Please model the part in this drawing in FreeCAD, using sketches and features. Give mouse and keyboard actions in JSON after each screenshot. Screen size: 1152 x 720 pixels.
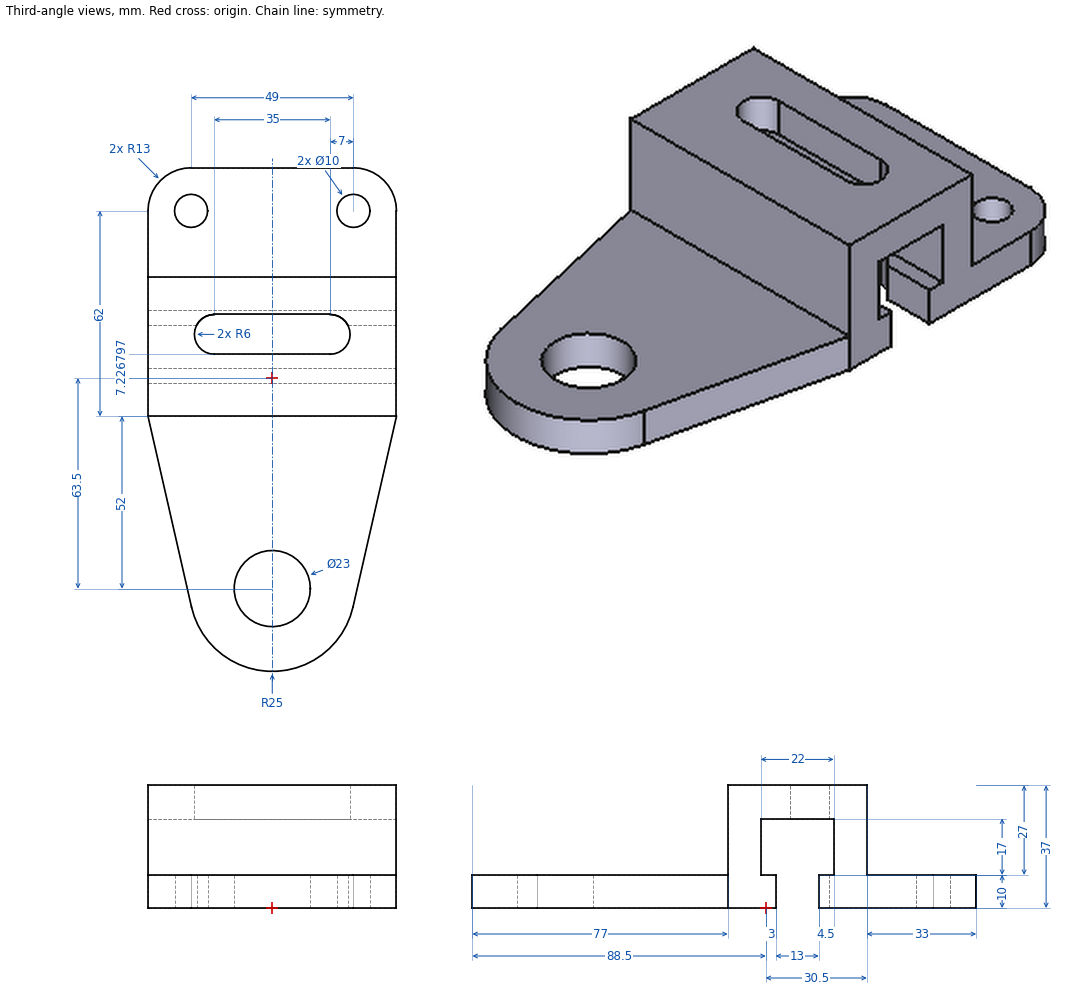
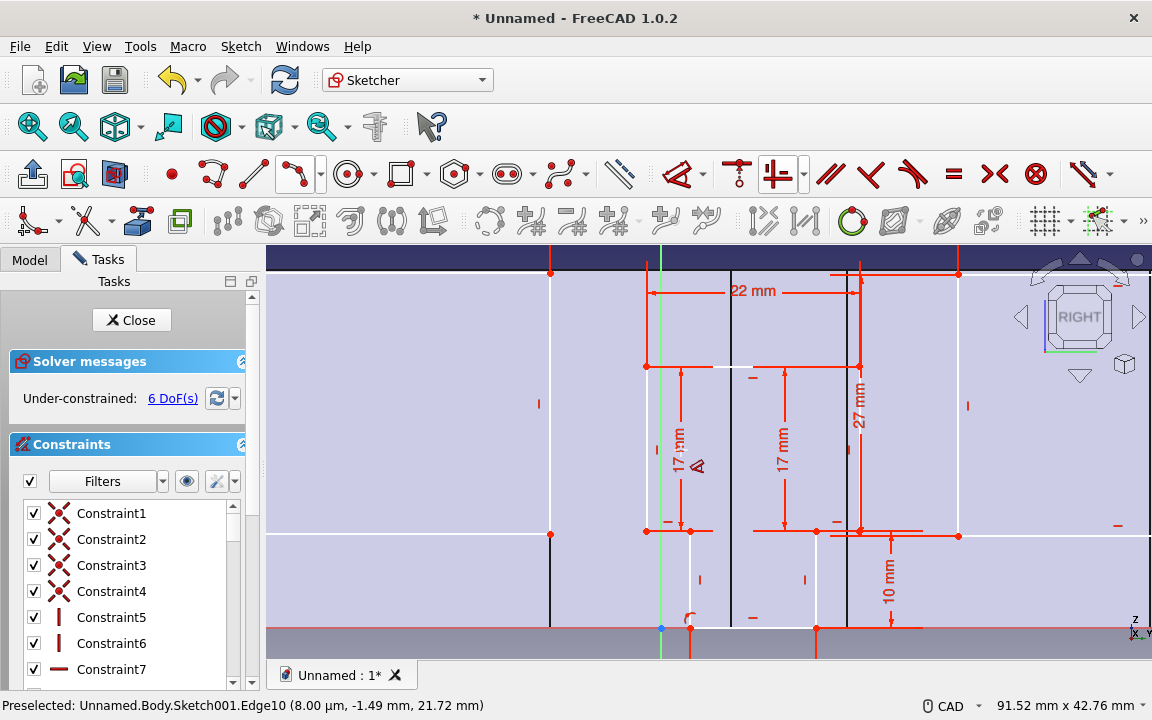
{"action": "scroll", "coordinate": [690, 628], "scroll_direction": "up", "scroll_amount": 2}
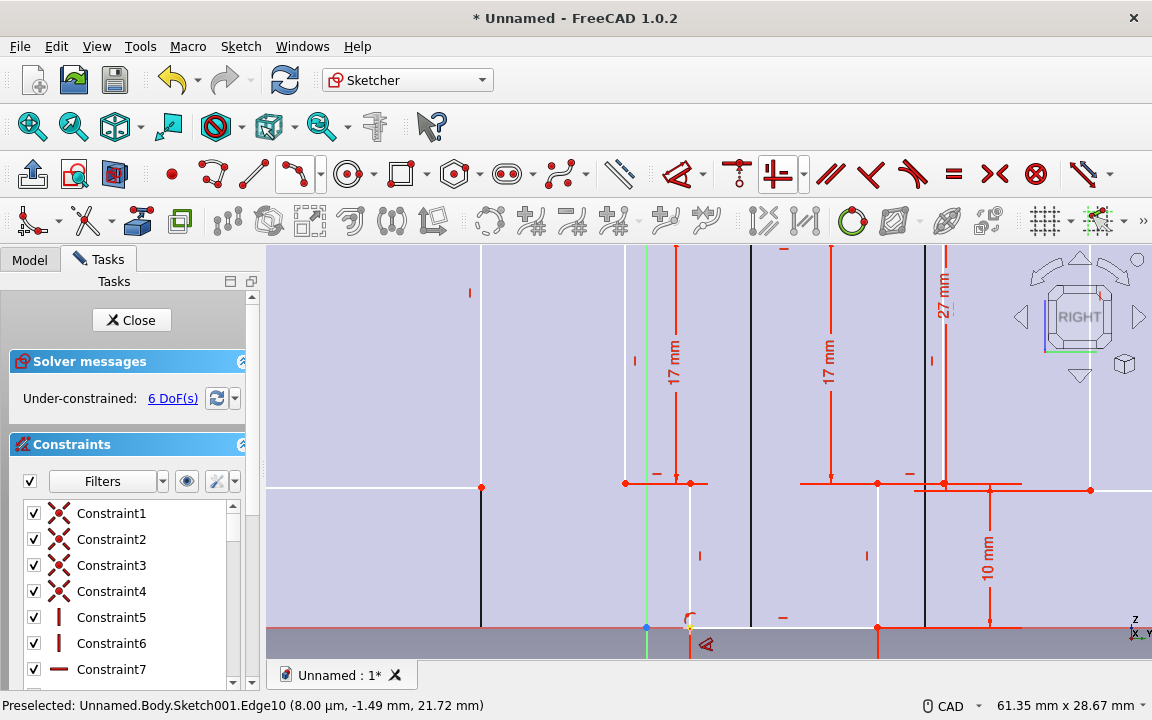
{"action": "left_click", "coordinate": [690, 628]}
{"action": "left_click", "coordinate": [668, 594]}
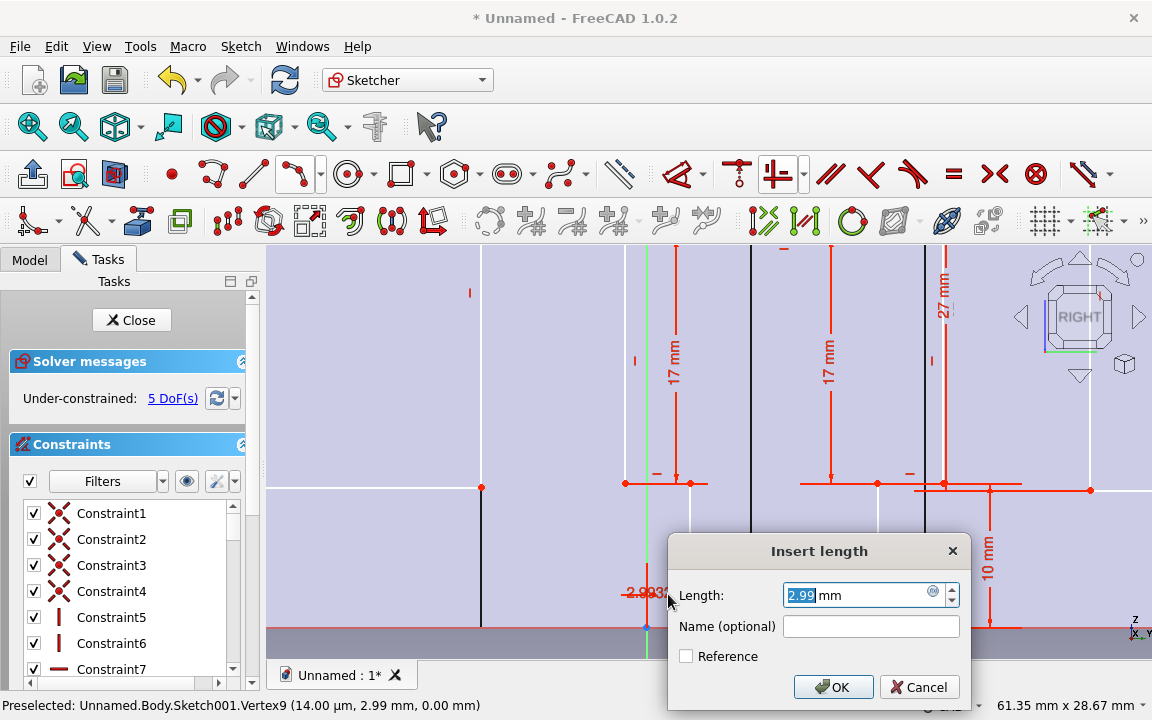
{"action": "type", "text": "3"}
{"action": "key", "text": "Return"}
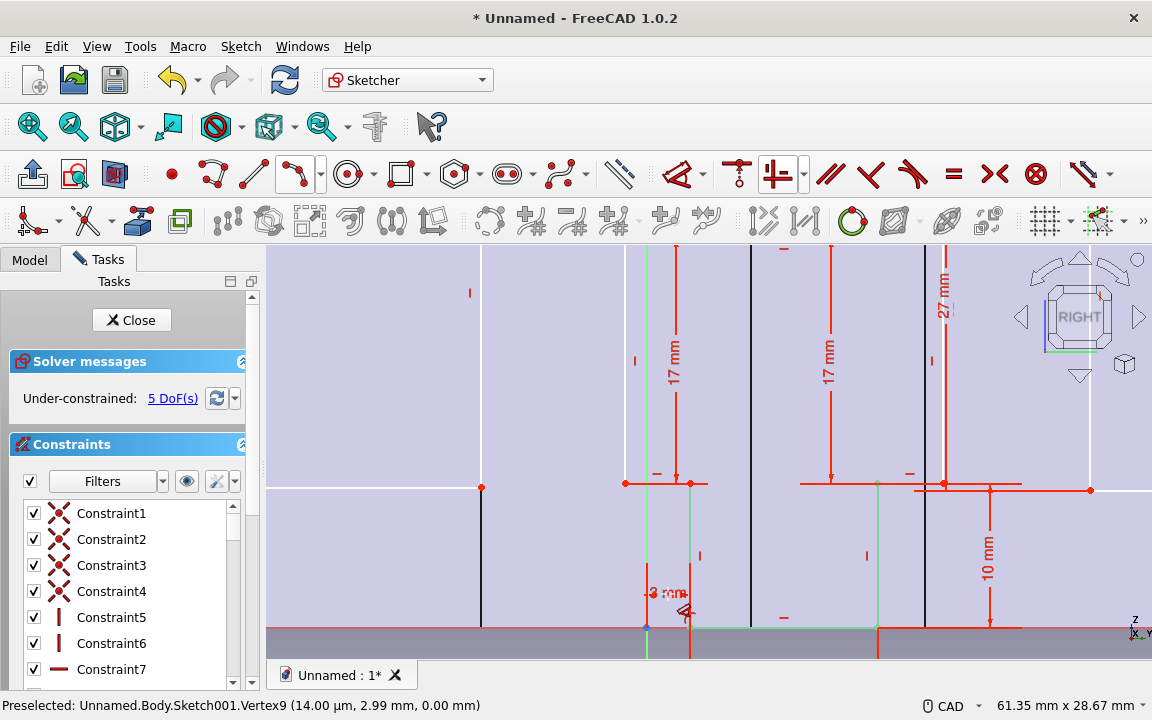
{"action": "left_click", "coordinate": [897, 484]}
{"action": "left_click", "coordinate": [911, 518]}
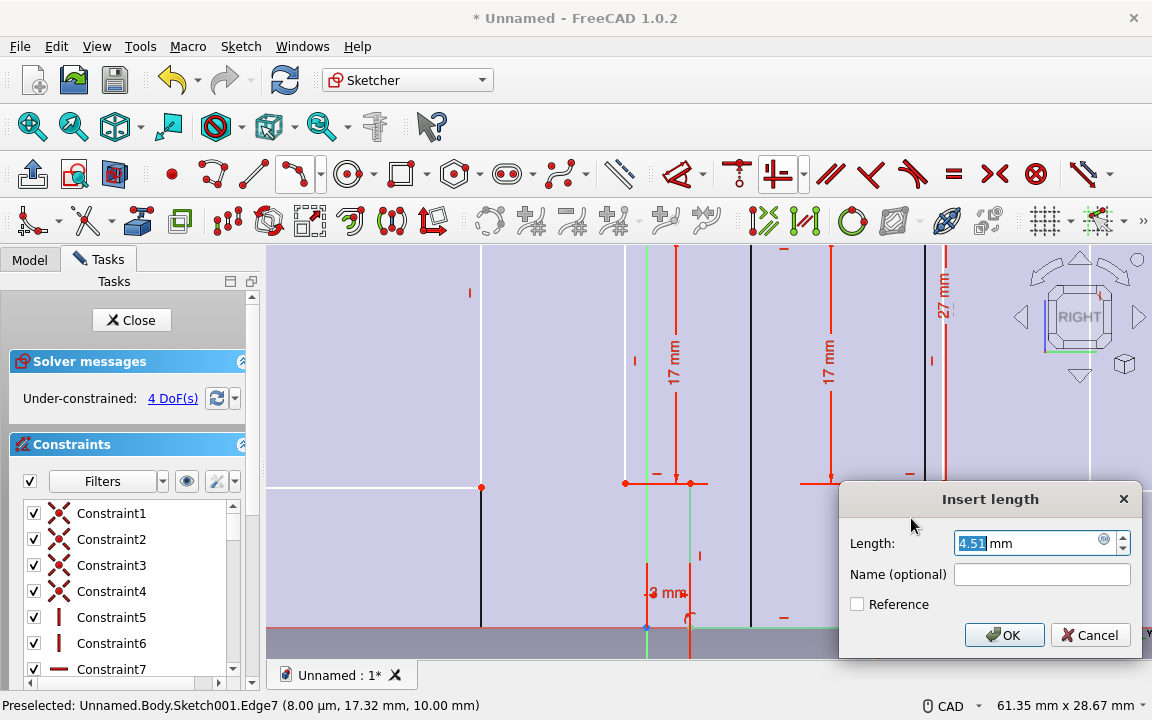
{"action": "type", "text": "4.5"}
{"action": "key", "text": "Return"}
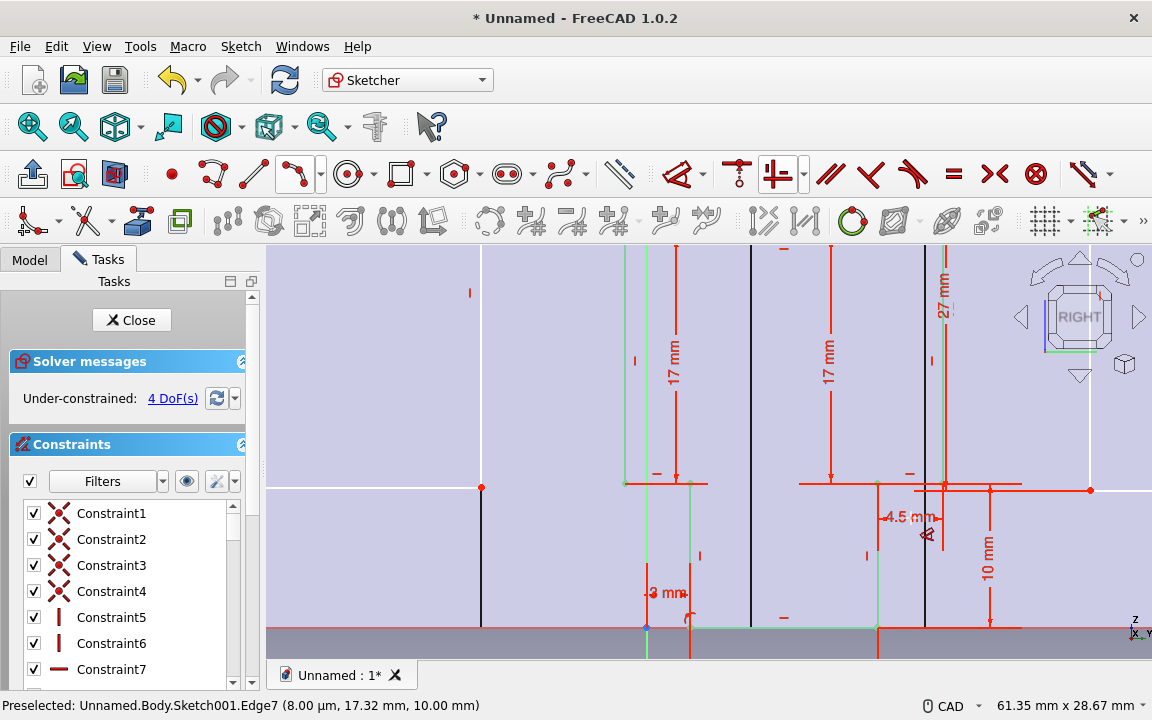
{"action": "scroll", "coordinate": [685, 475], "scroll_direction": "down", "scroll_amount": 8}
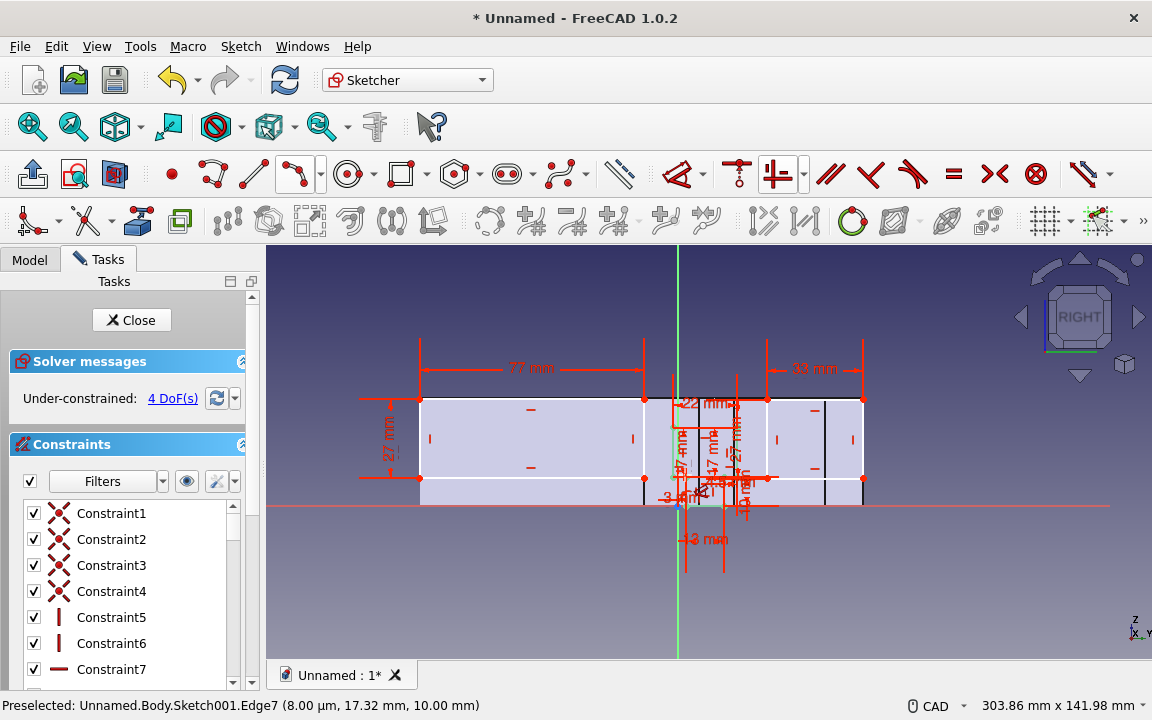
{"action": "left_click", "coordinate": [767, 400]}
{"action": "left_click", "coordinate": [801, 453]}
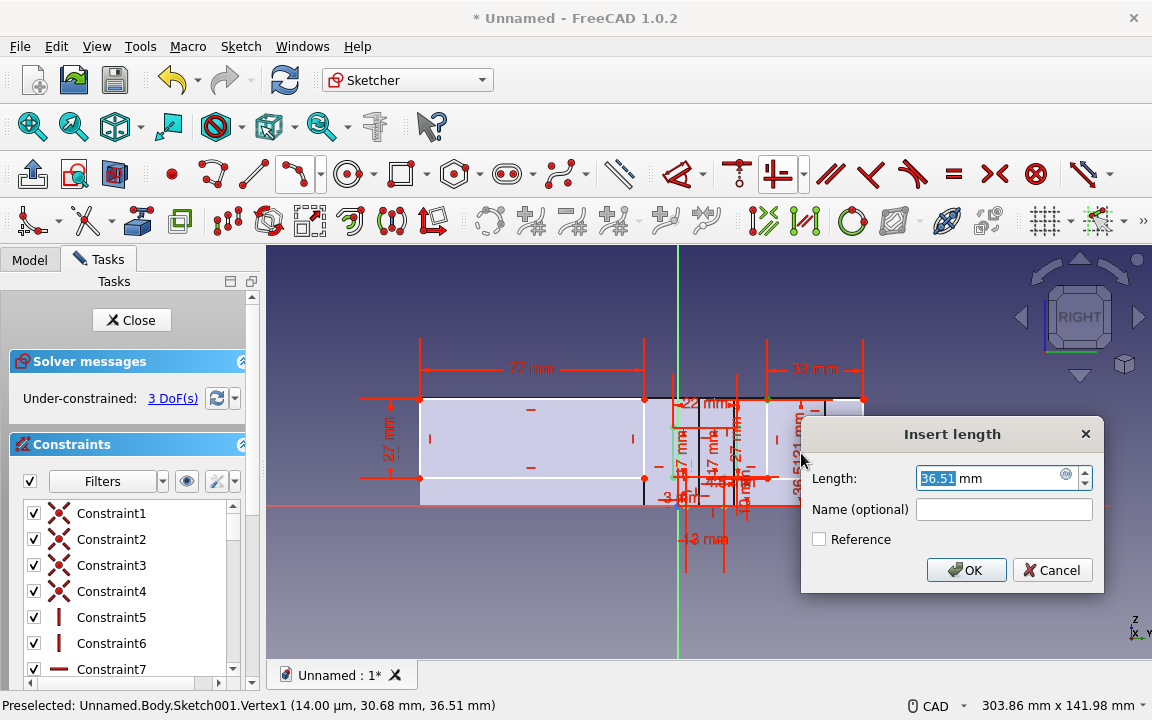
{"action": "type", "text": "37"}
{"action": "key", "text": "Return"}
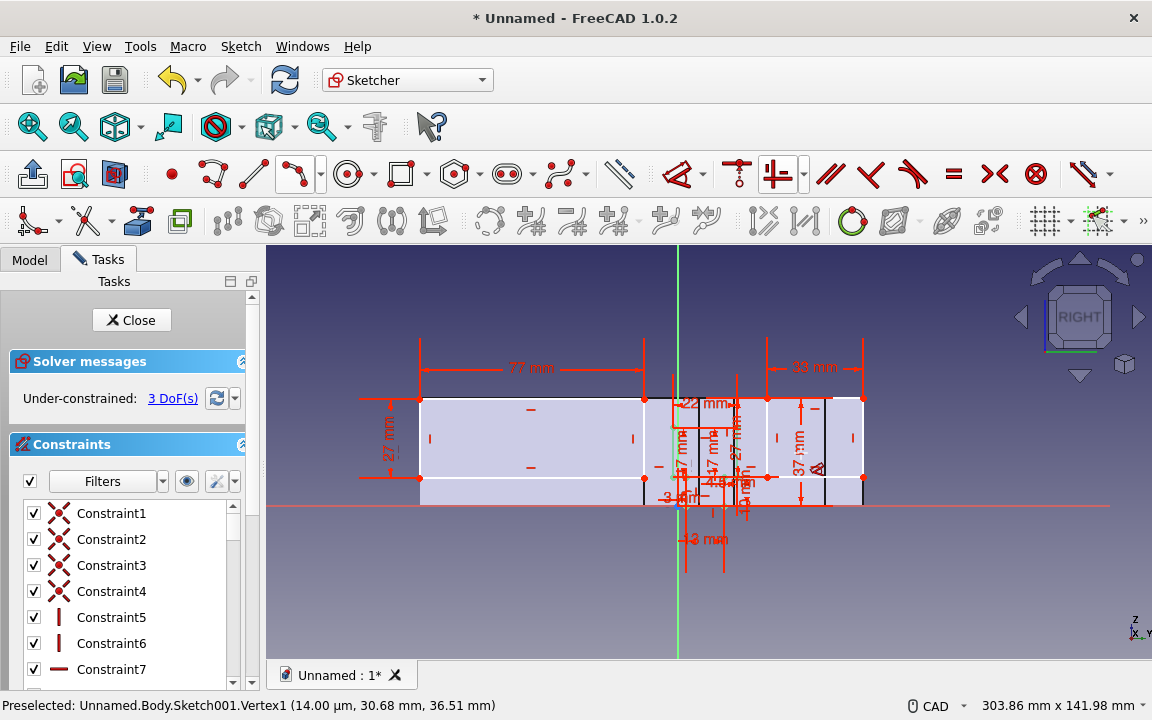
{"action": "left_click", "coordinate": [420, 399]}
{"action": "left_click", "coordinate": [386, 453]}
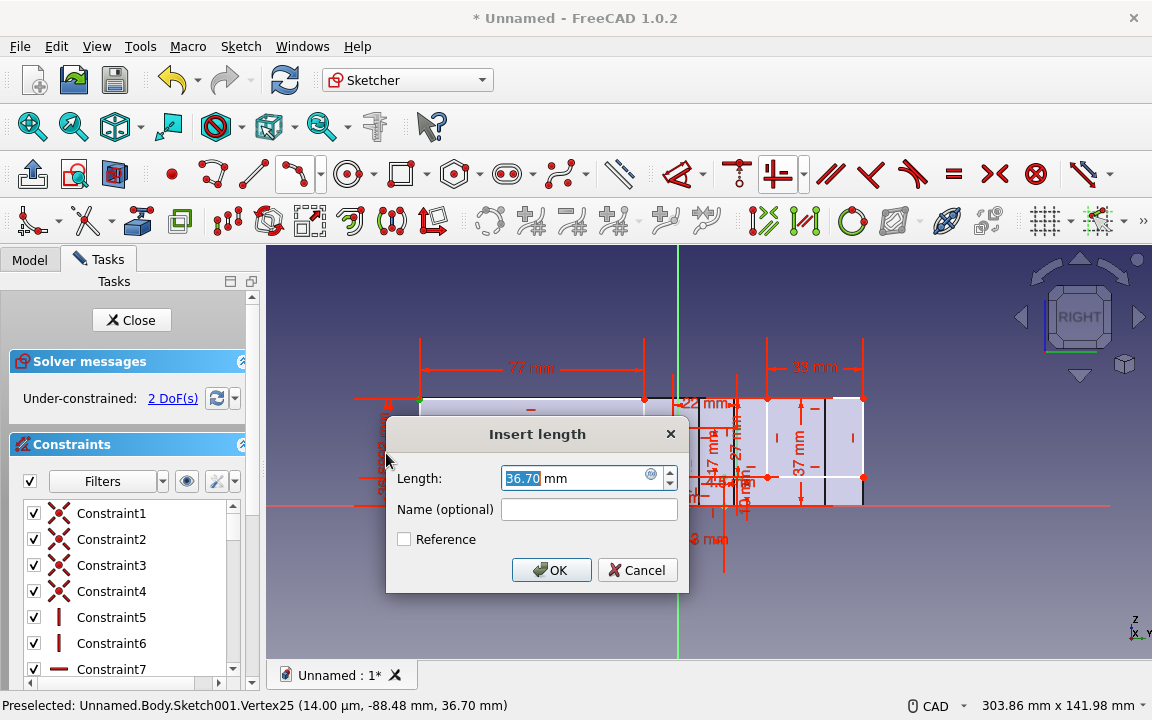
{"action": "type", "text": "37"}
{"action": "key", "text": "Return"}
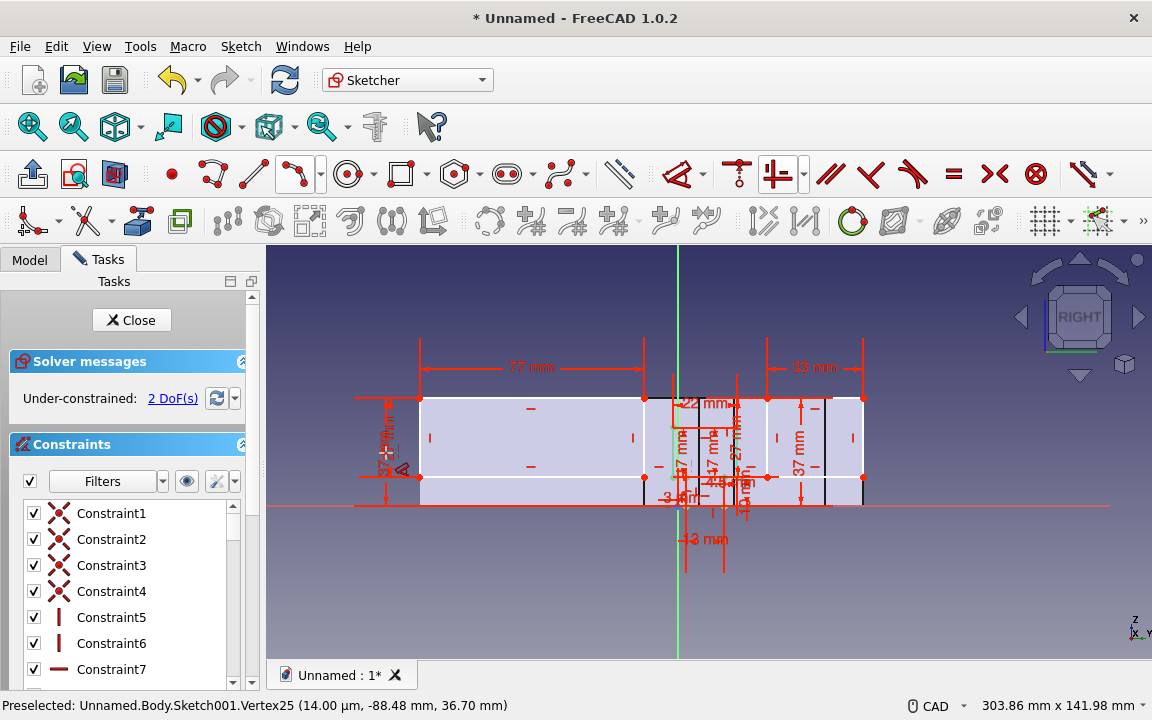
{"action": "left_click", "coordinate": [767, 398]}
{"action": "left_click", "coordinate": [722, 364]}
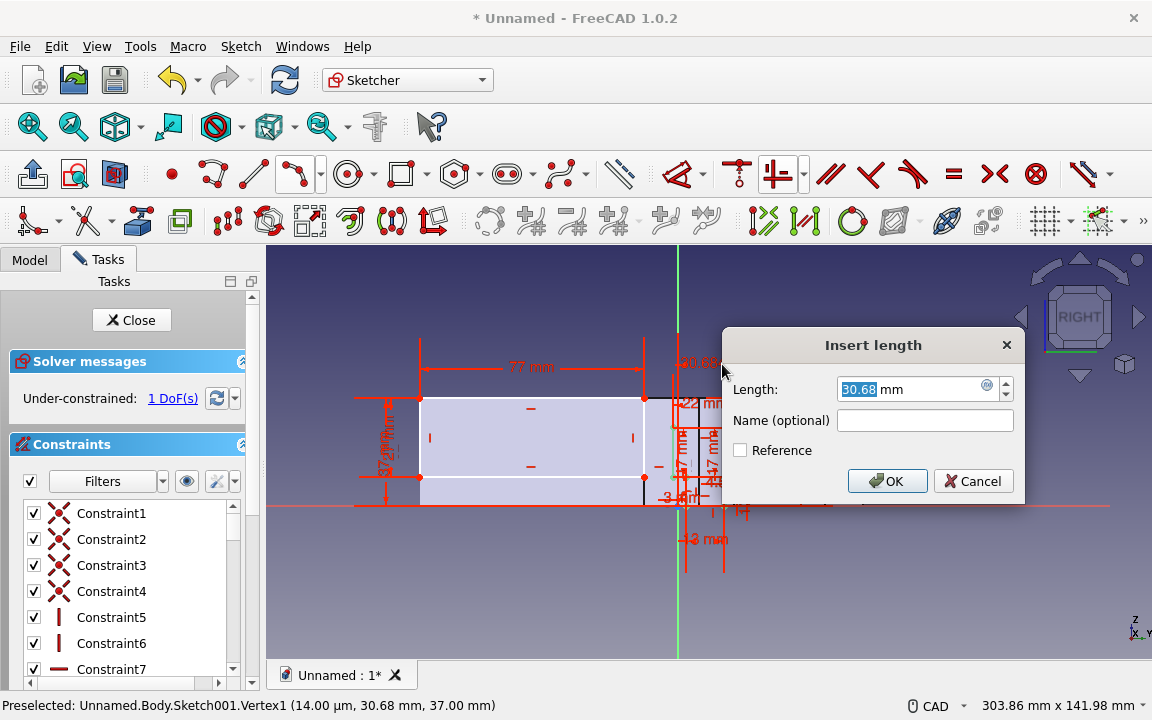
{"action": "type", "text": "30.5"}
{"action": "key", "text": "Return"}